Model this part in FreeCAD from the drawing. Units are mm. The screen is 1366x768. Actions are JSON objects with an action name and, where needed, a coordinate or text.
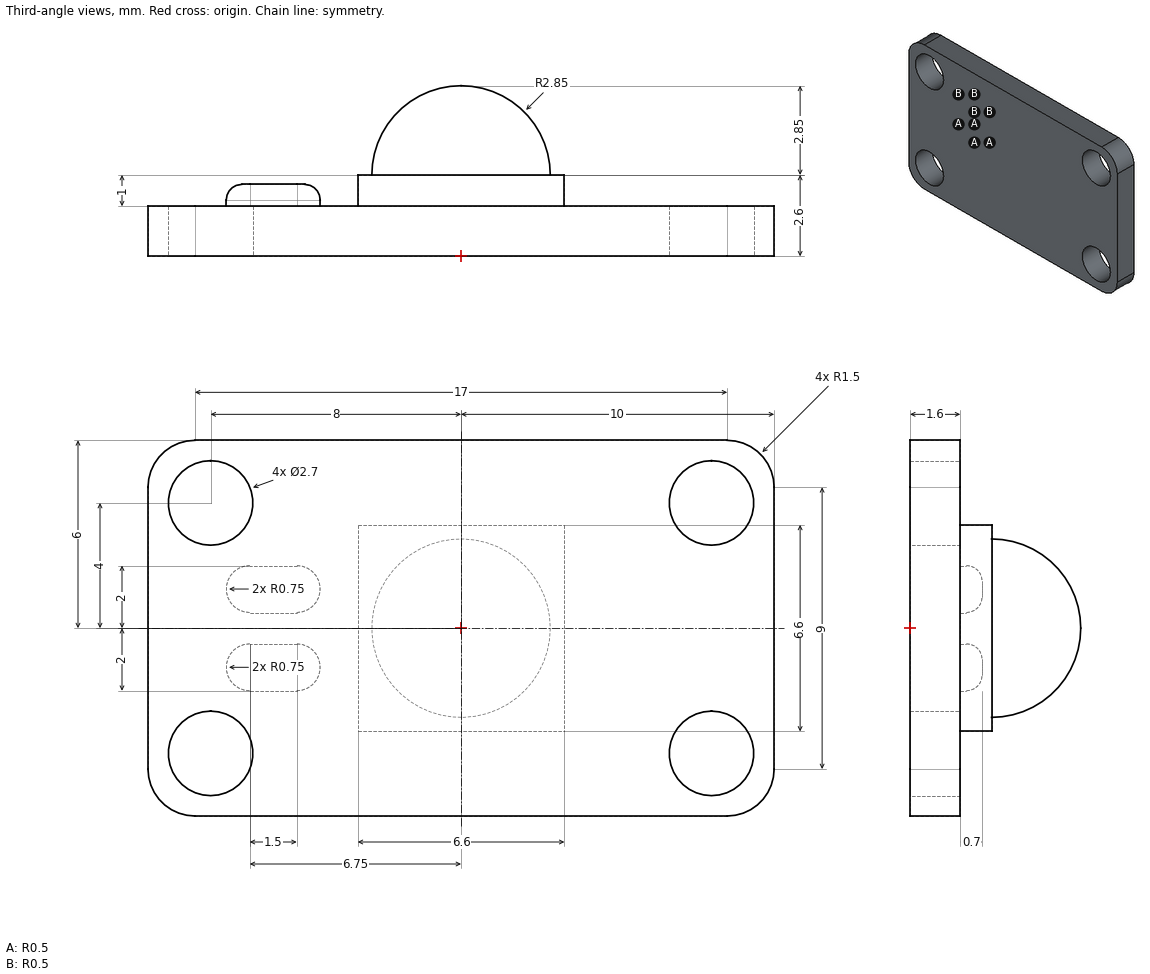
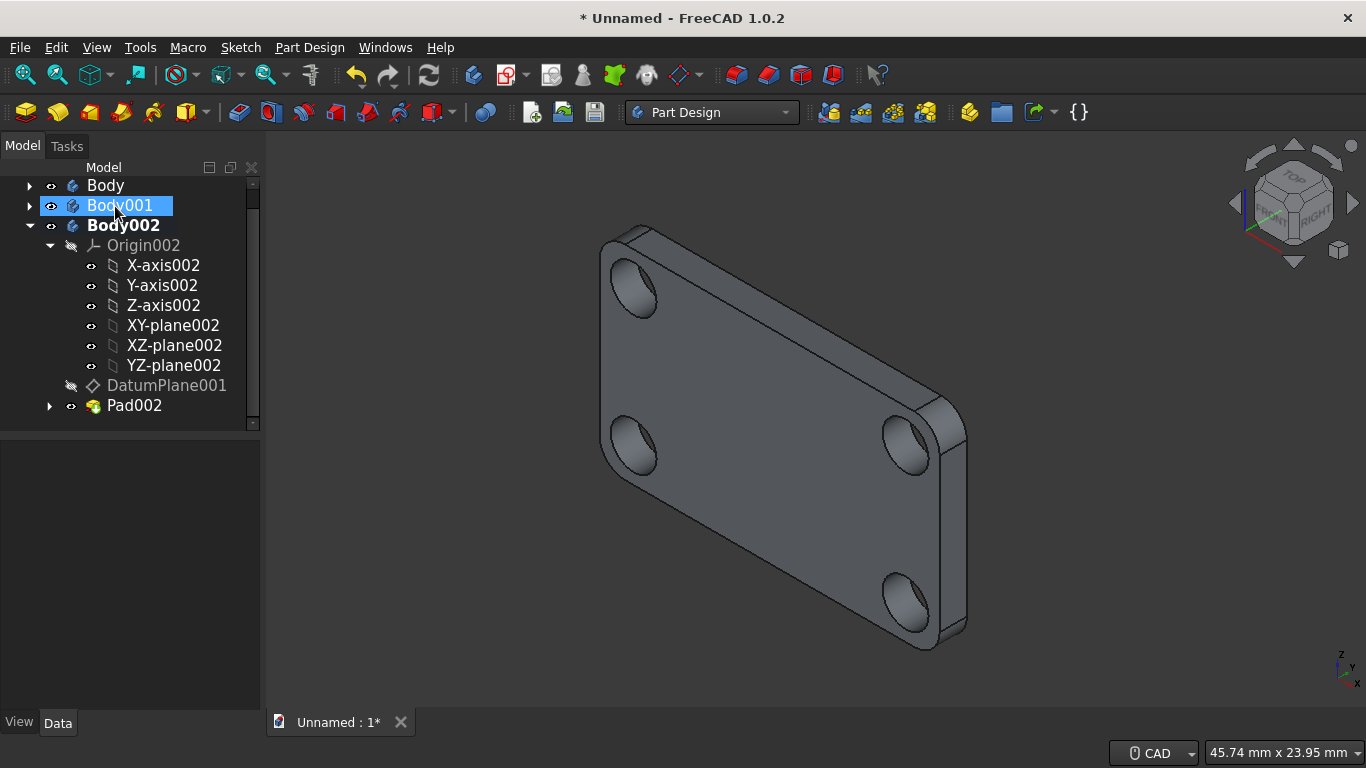
{"action": "key", "text": "2"}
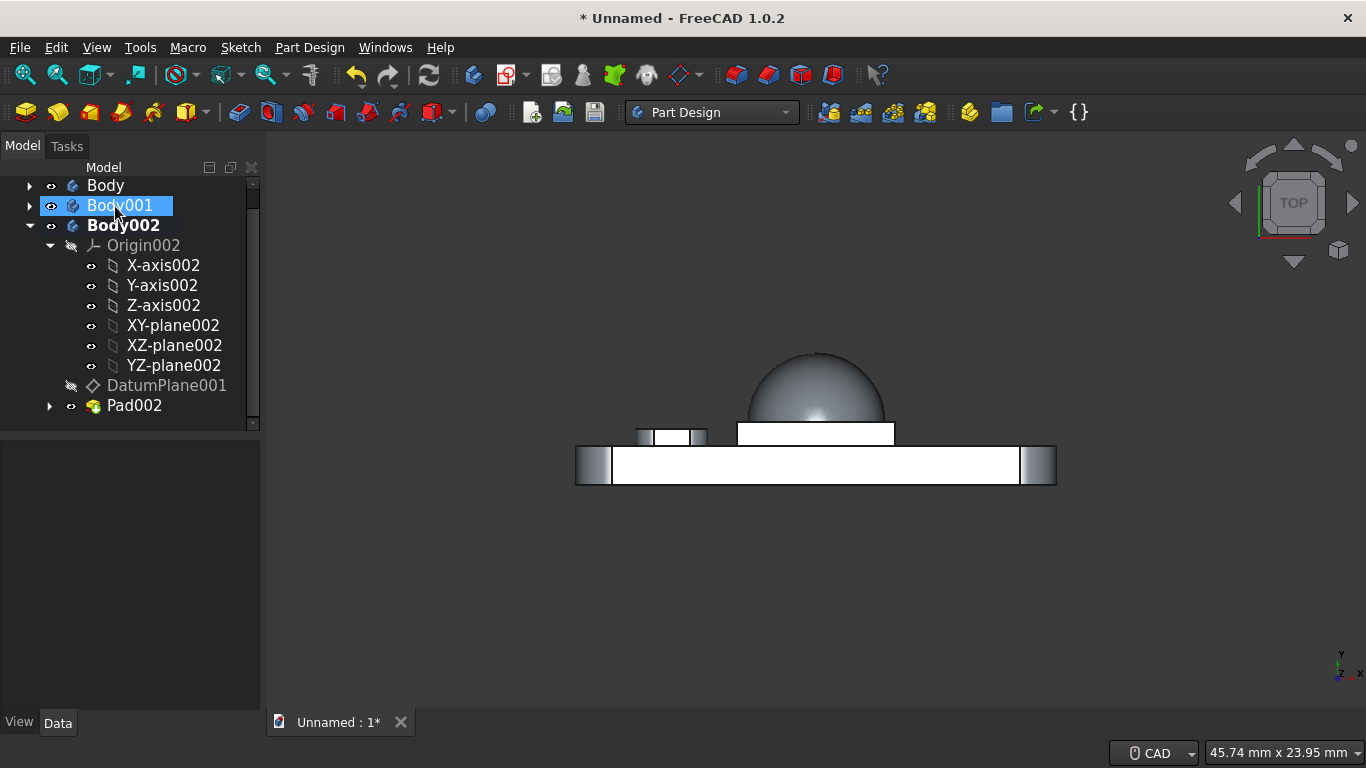
{"action": "left_click", "coordinate": [26, 76]}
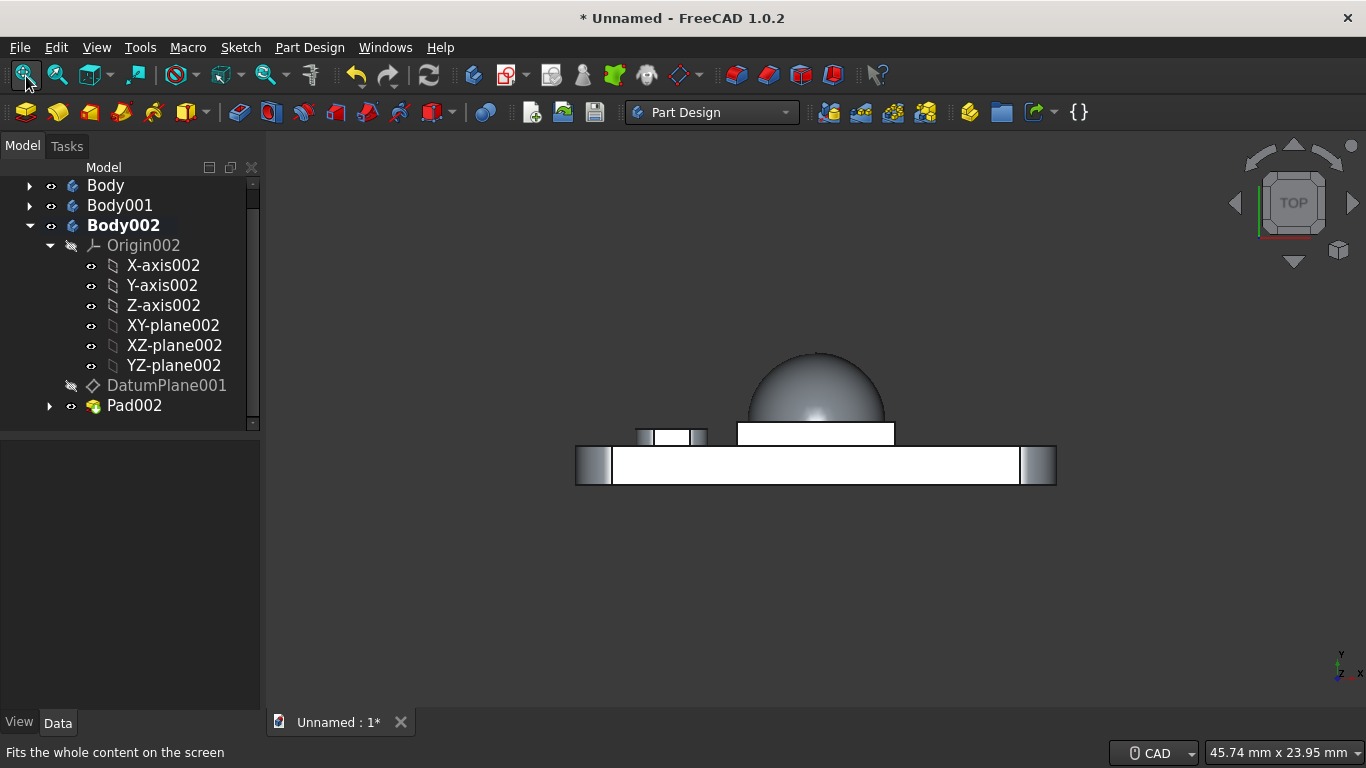
{"action": "key", "text": "1"}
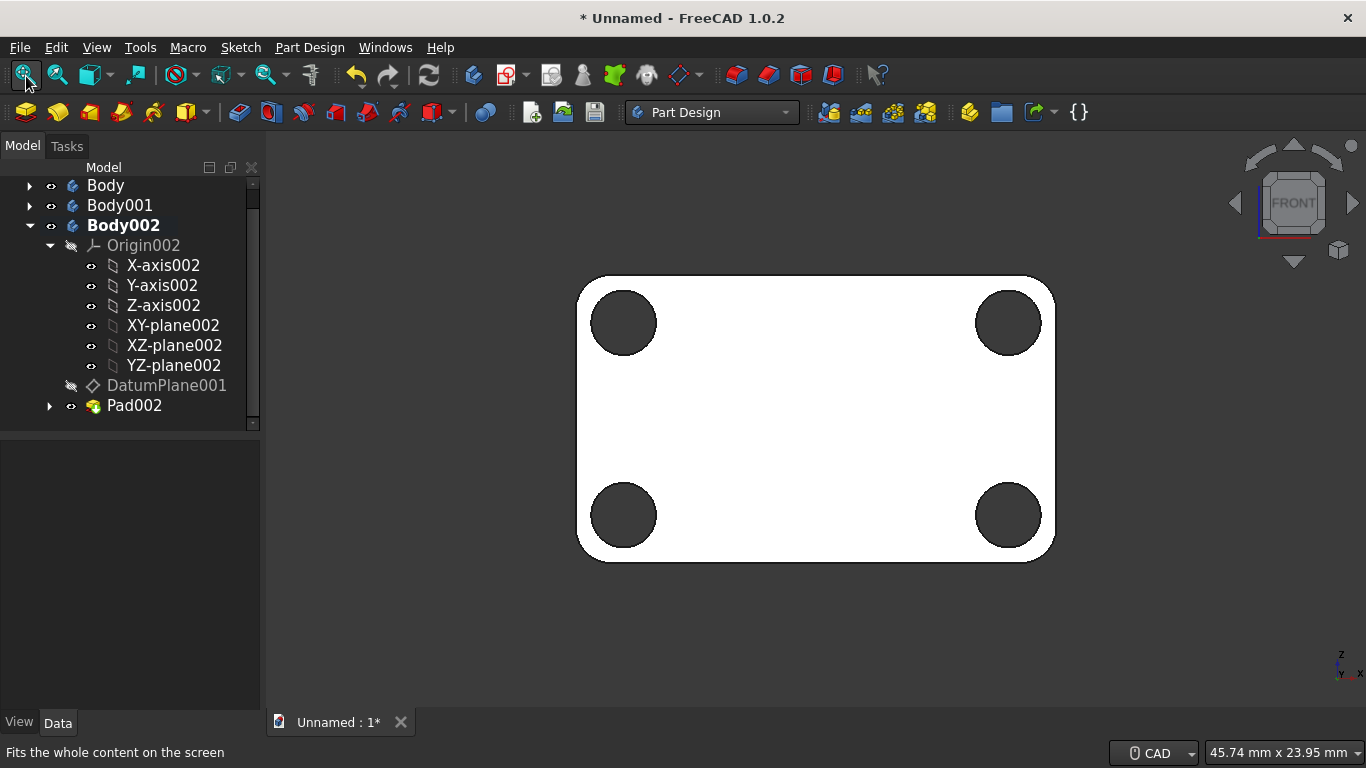
{"action": "left_click", "coordinate": [26, 76]}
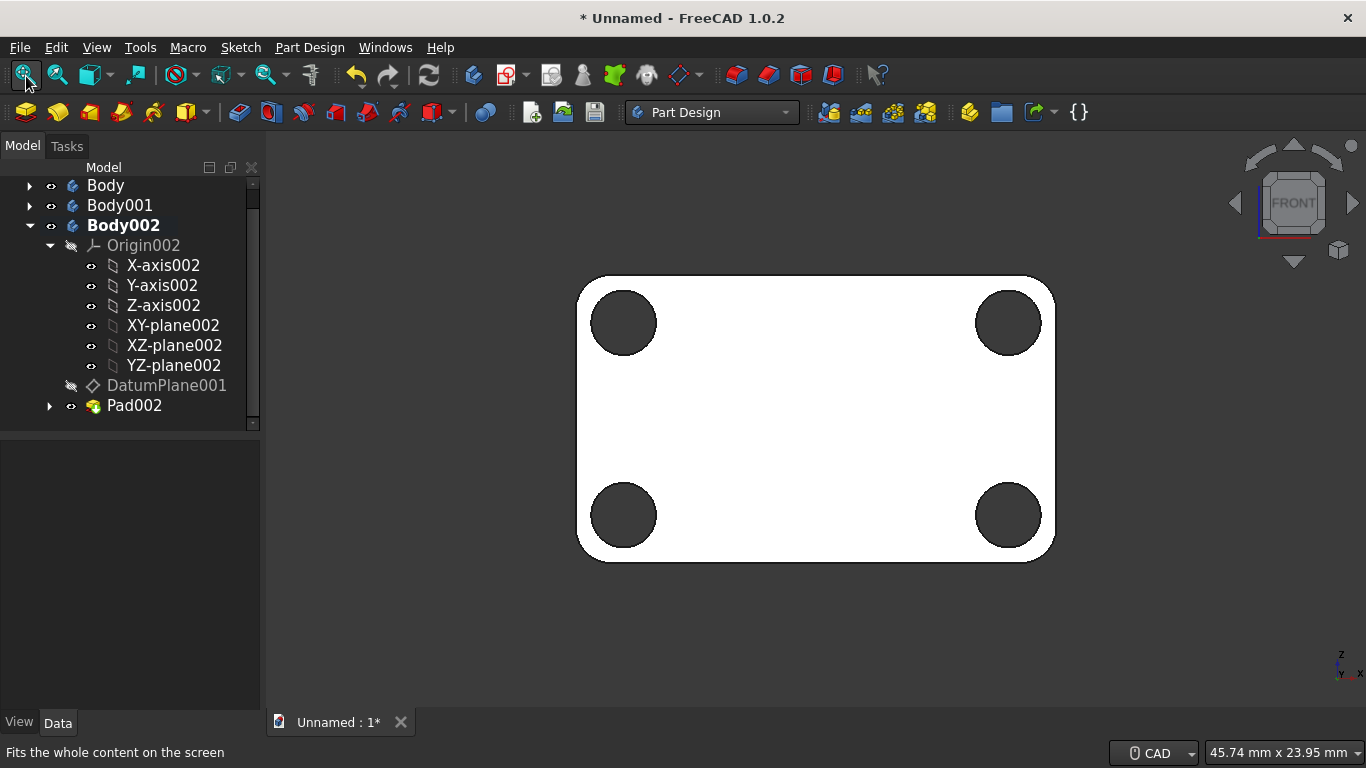
{"action": "key", "text": "3"}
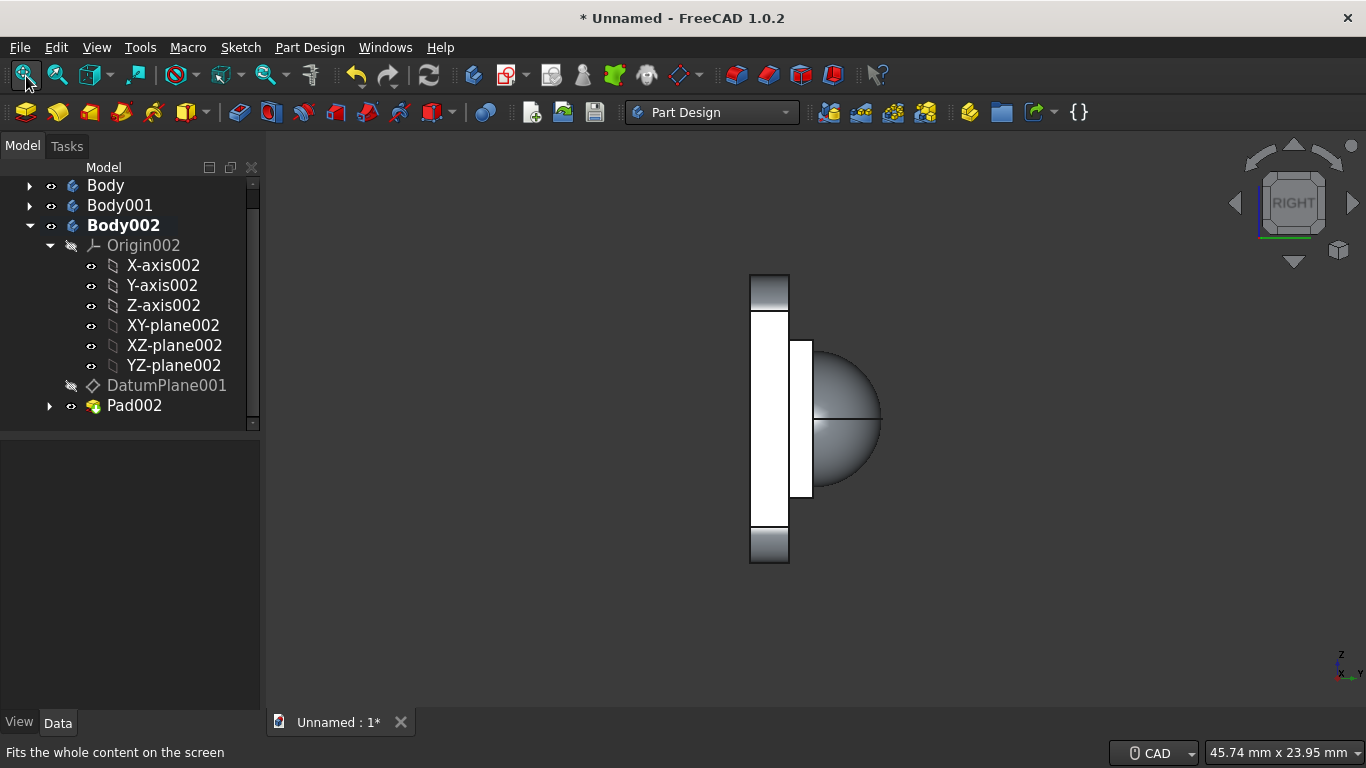
{"action": "left_click", "coordinate": [26, 76]}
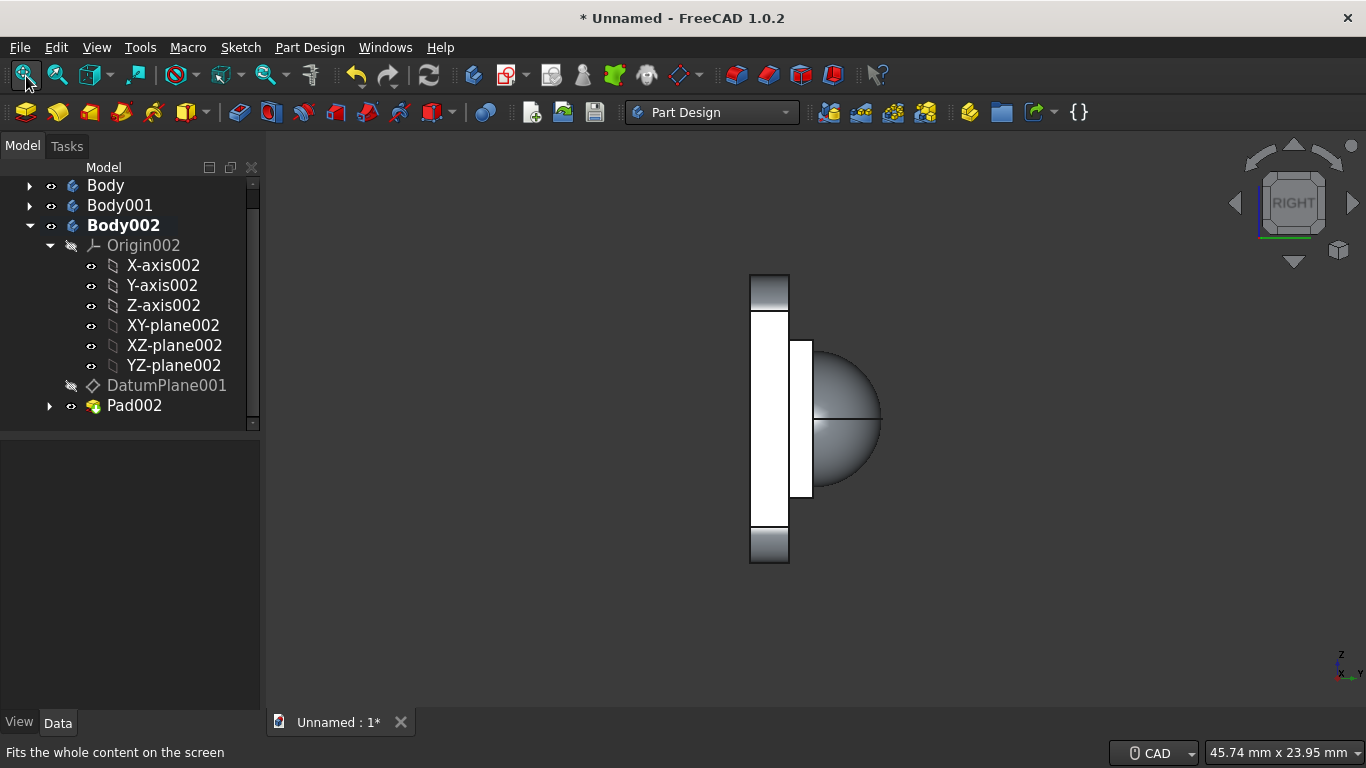
{"action": "key", "text": "5"}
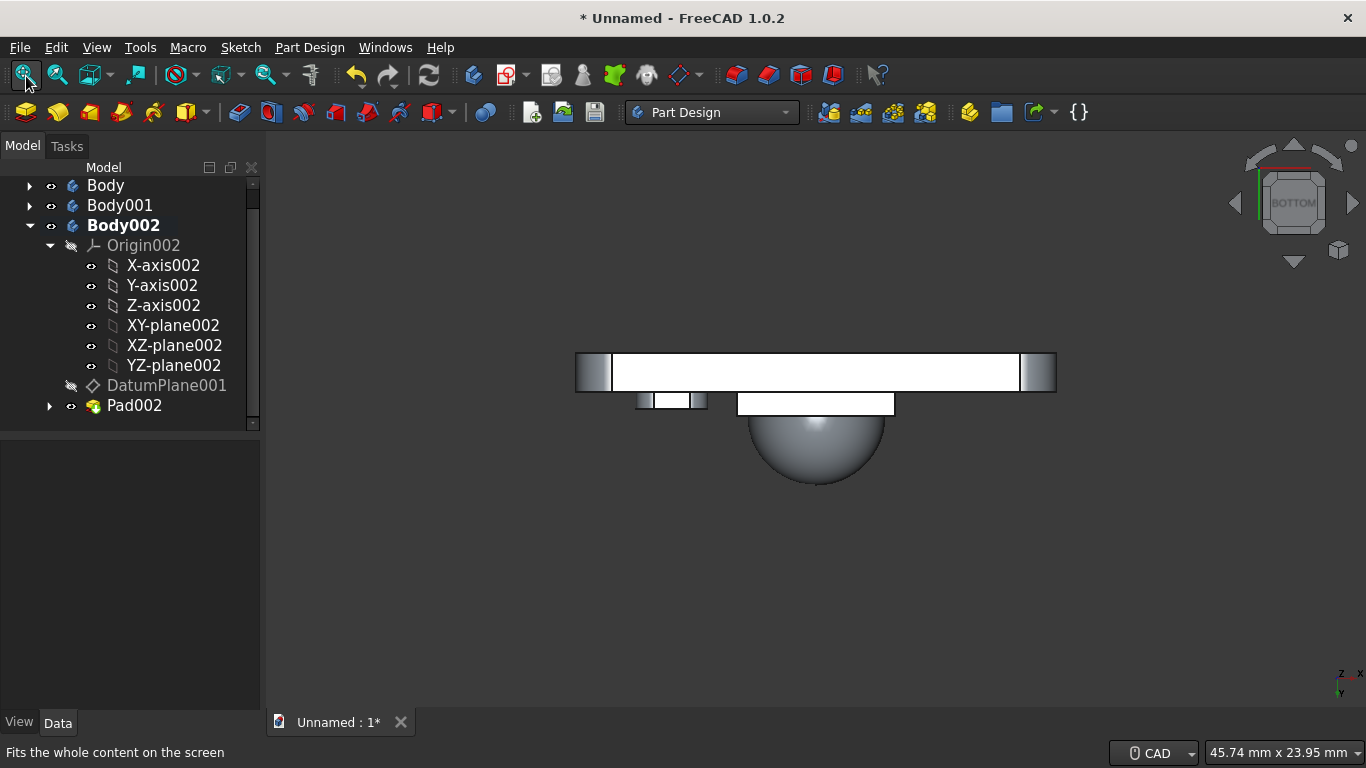
{"action": "left_click", "coordinate": [26, 76]}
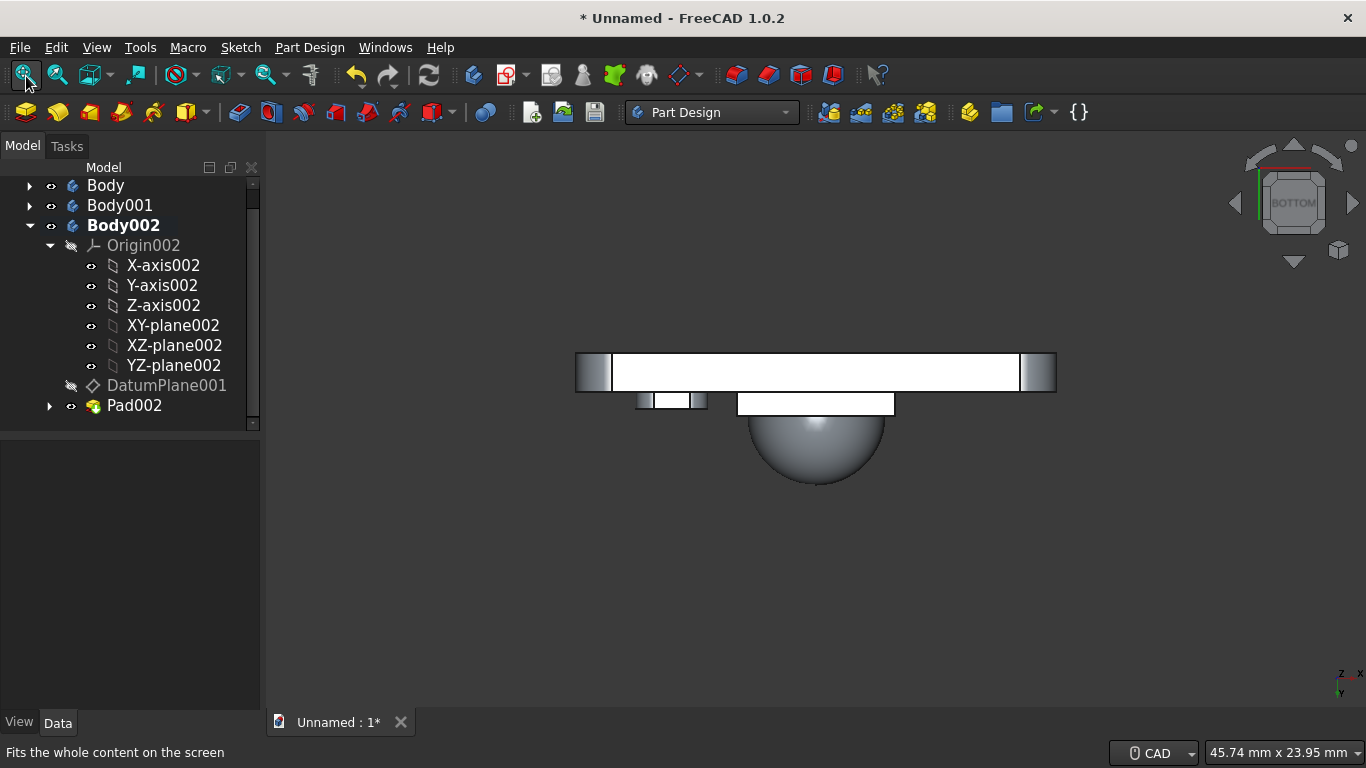
{"action": "key", "text": "4"}